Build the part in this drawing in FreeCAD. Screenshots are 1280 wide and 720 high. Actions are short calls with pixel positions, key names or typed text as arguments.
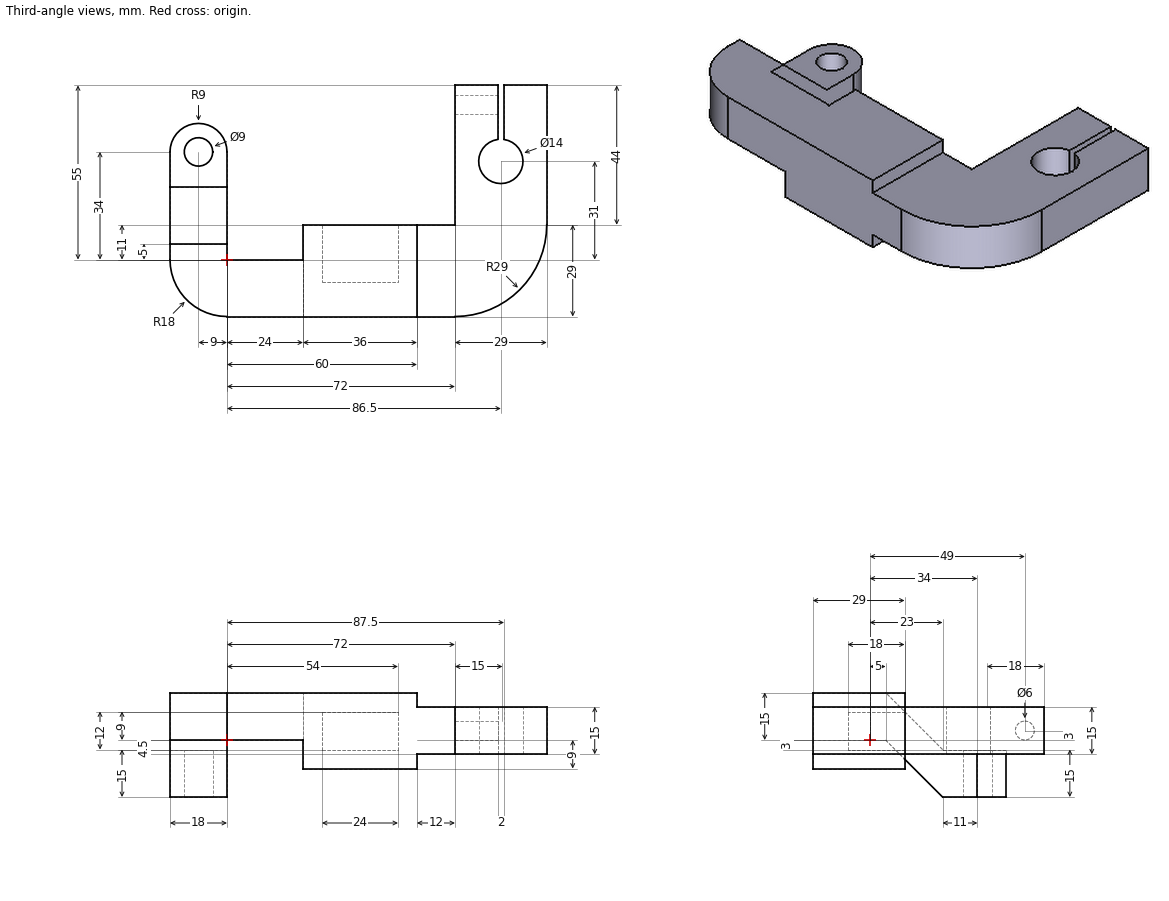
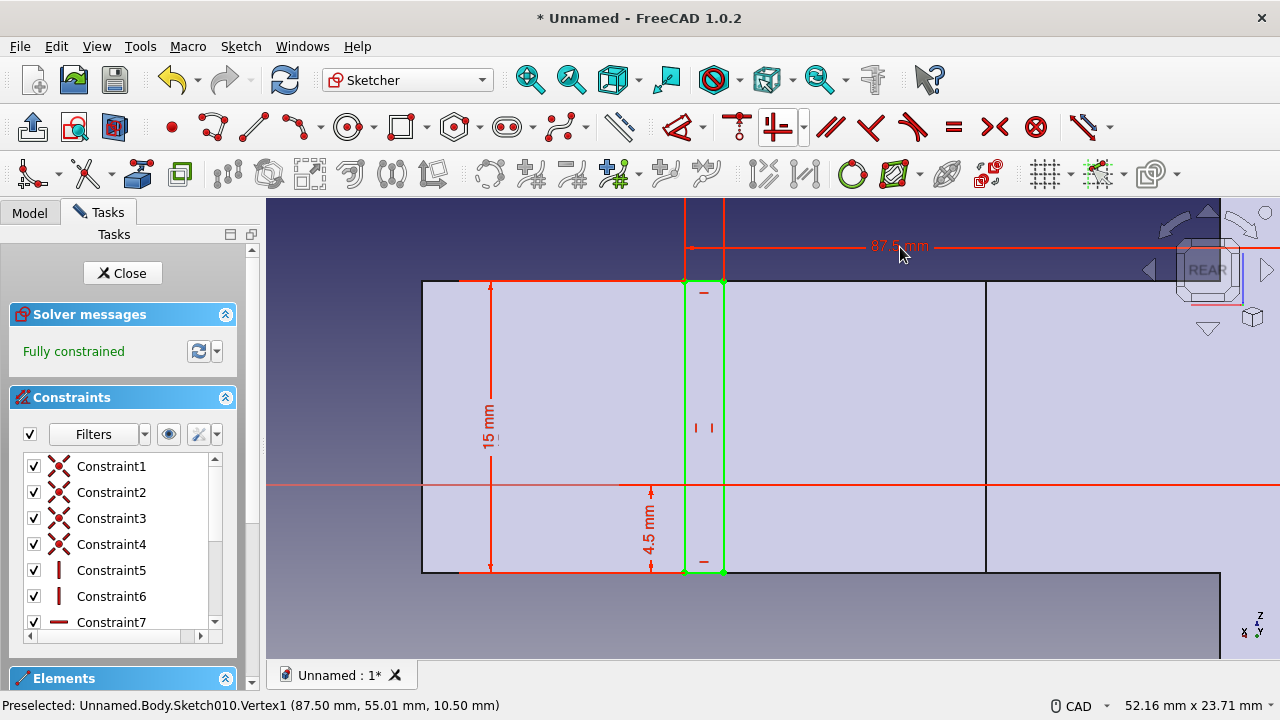
click(123, 273)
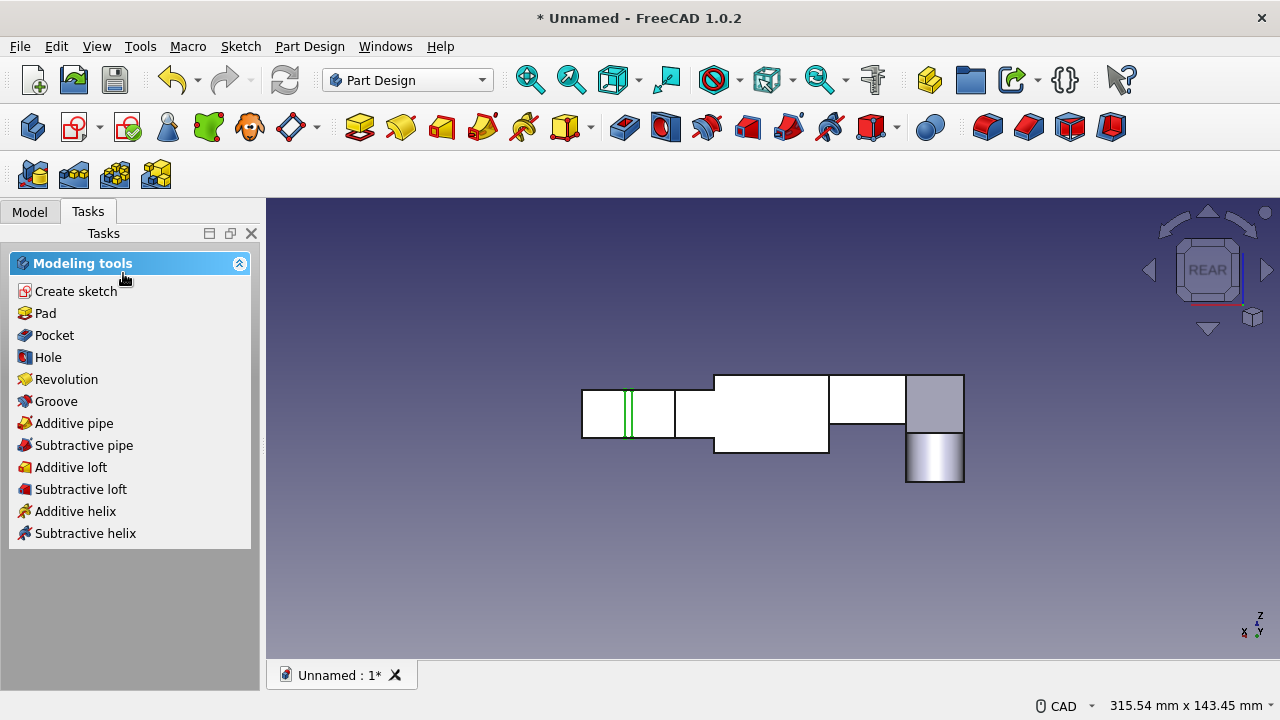
click(625, 128)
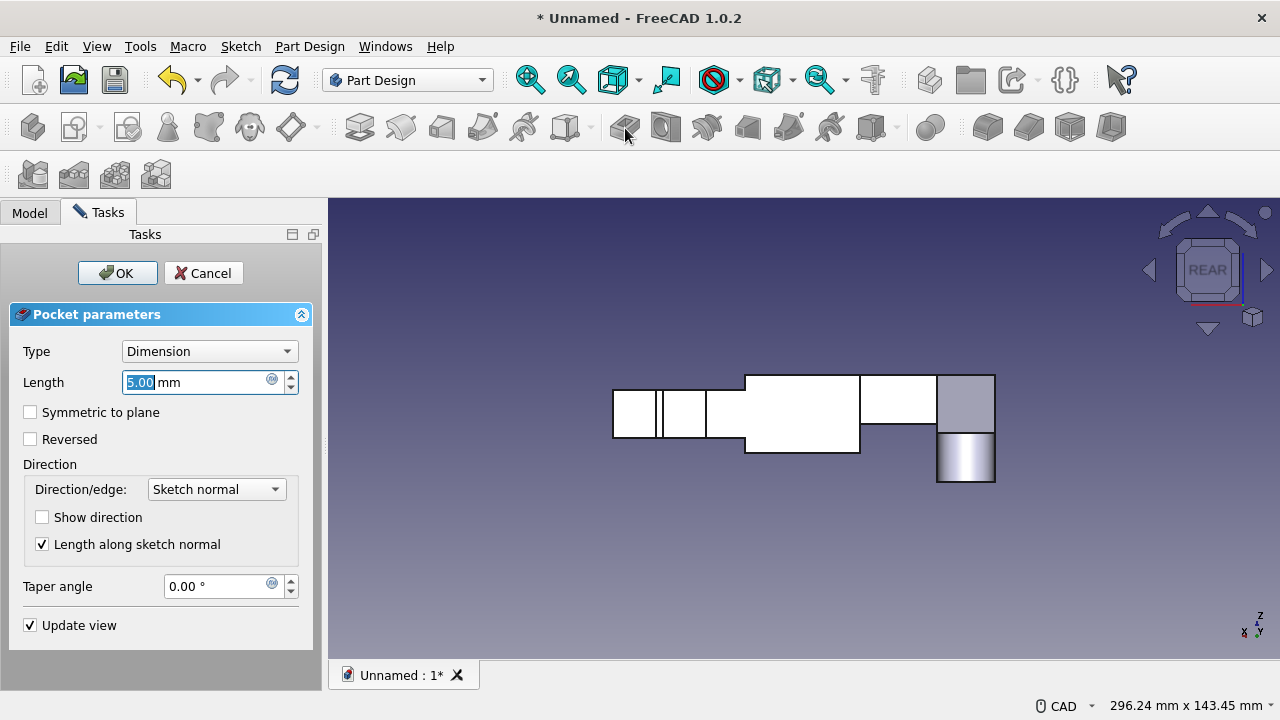
text(18)
key(Tab)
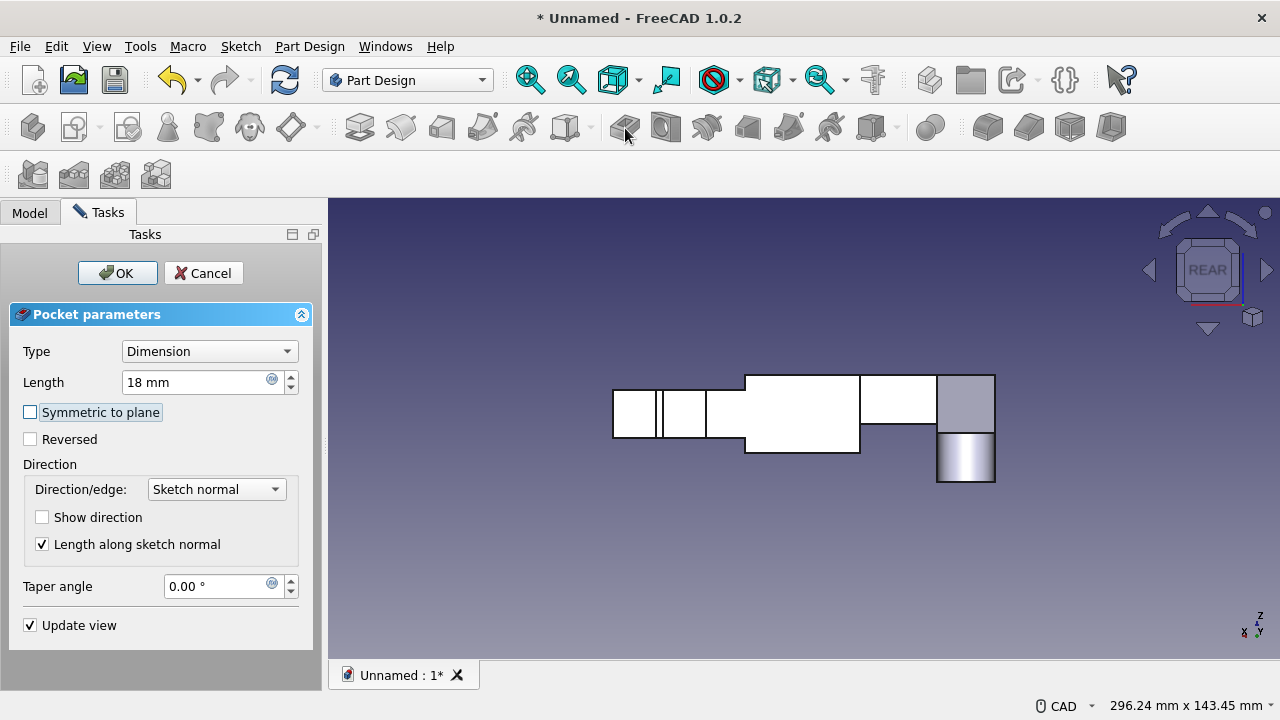
click(118, 273)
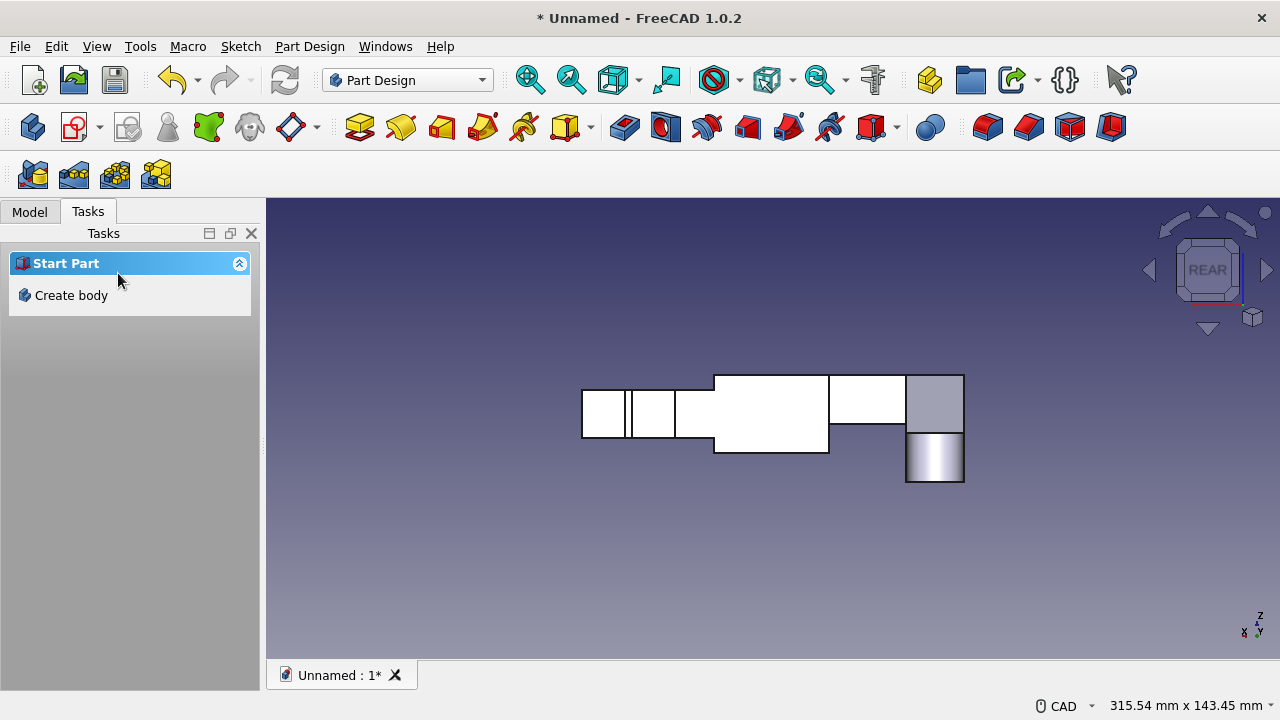
click(531, 80)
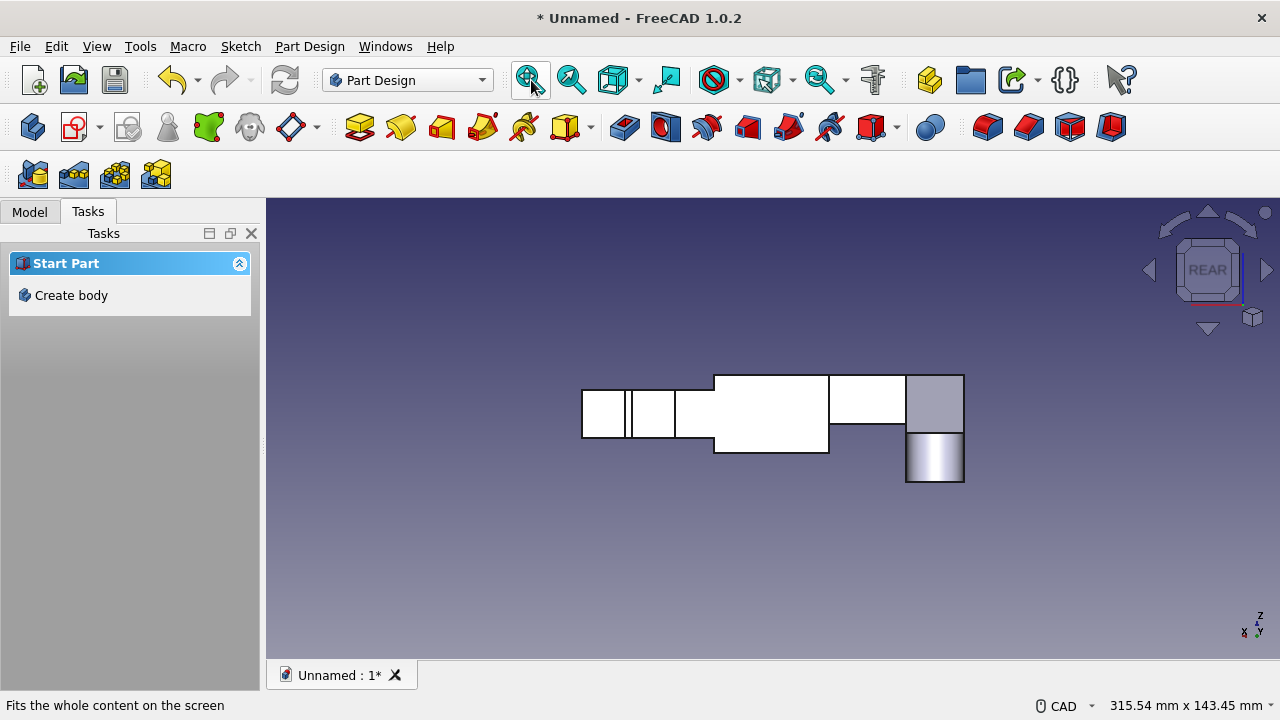
key(6)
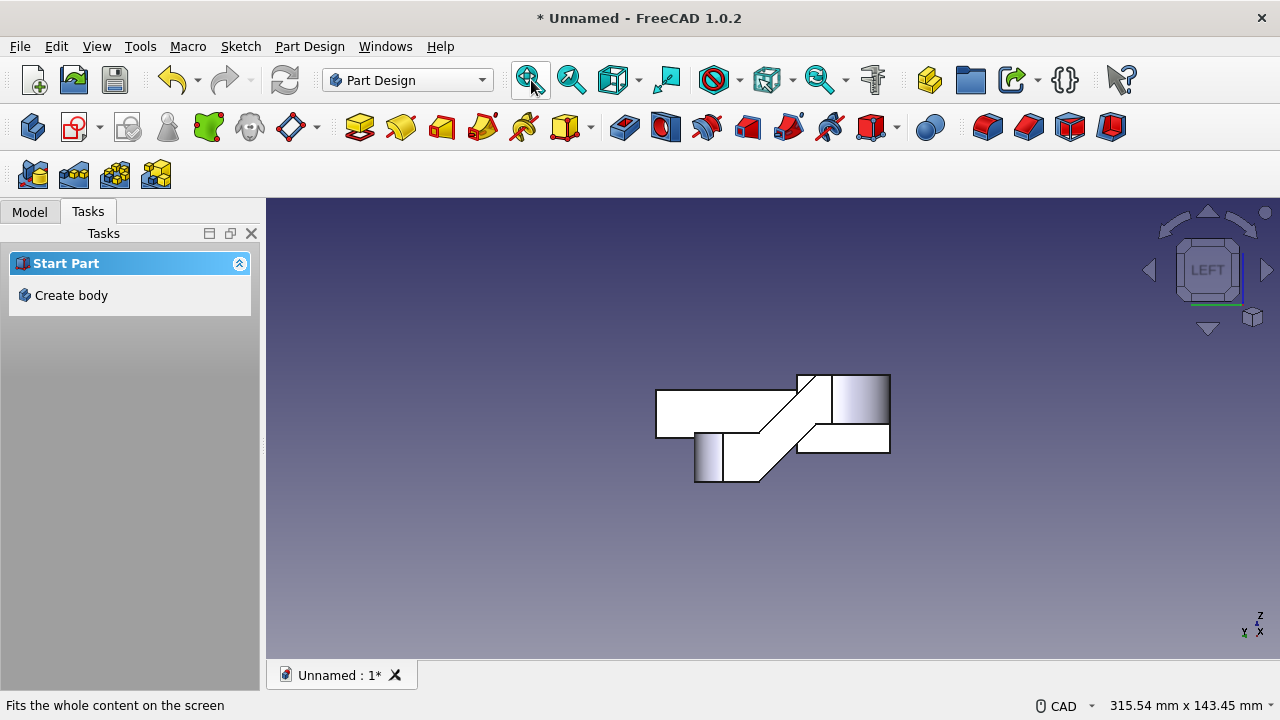
click(531, 80)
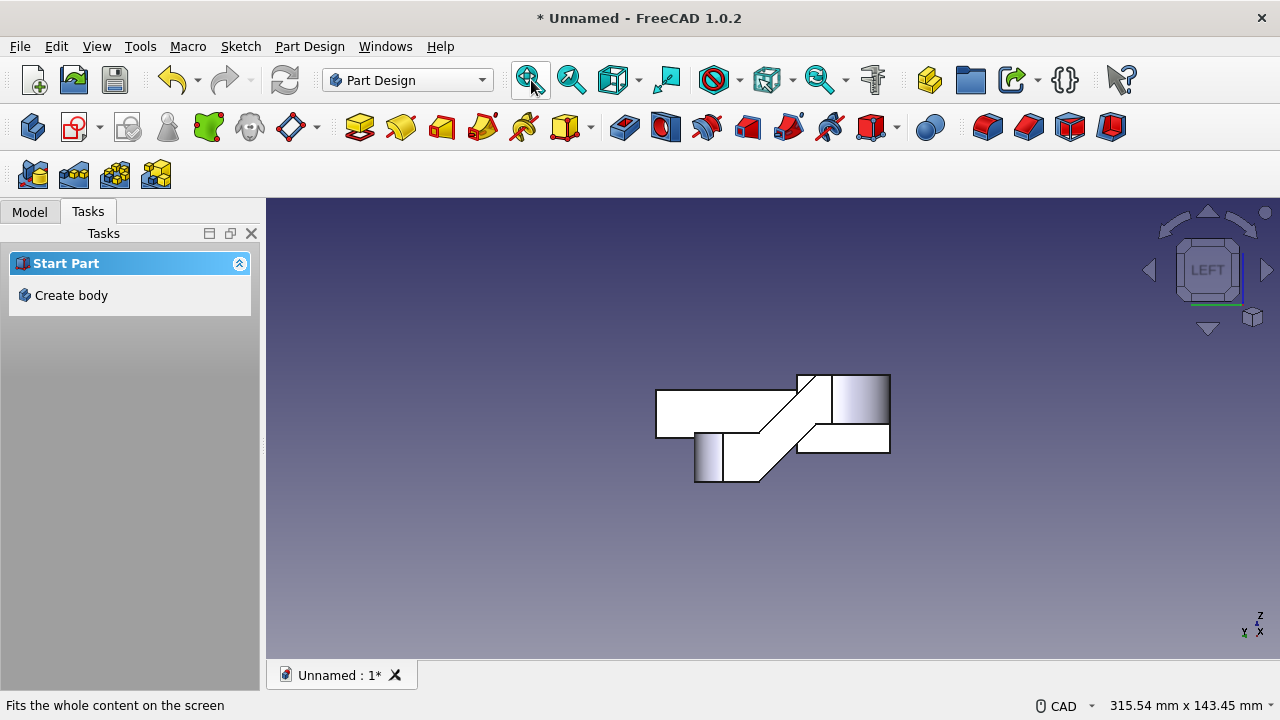
click(686, 413)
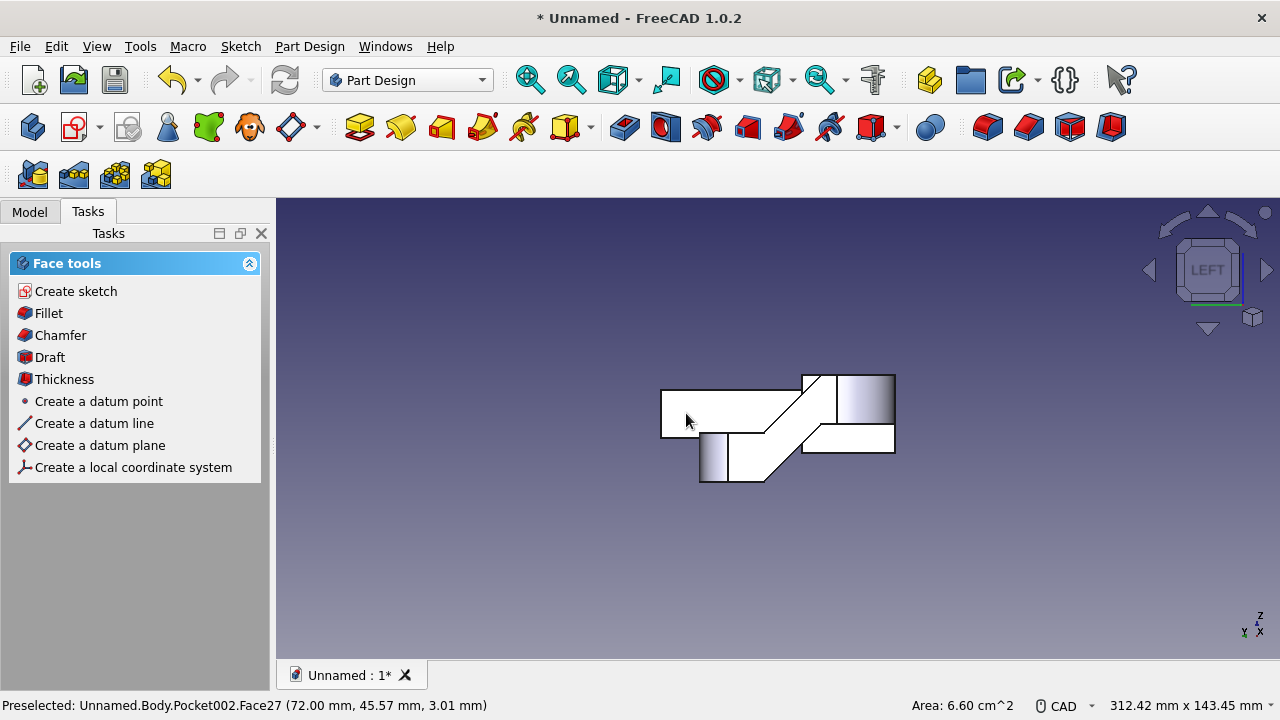
click(74, 128)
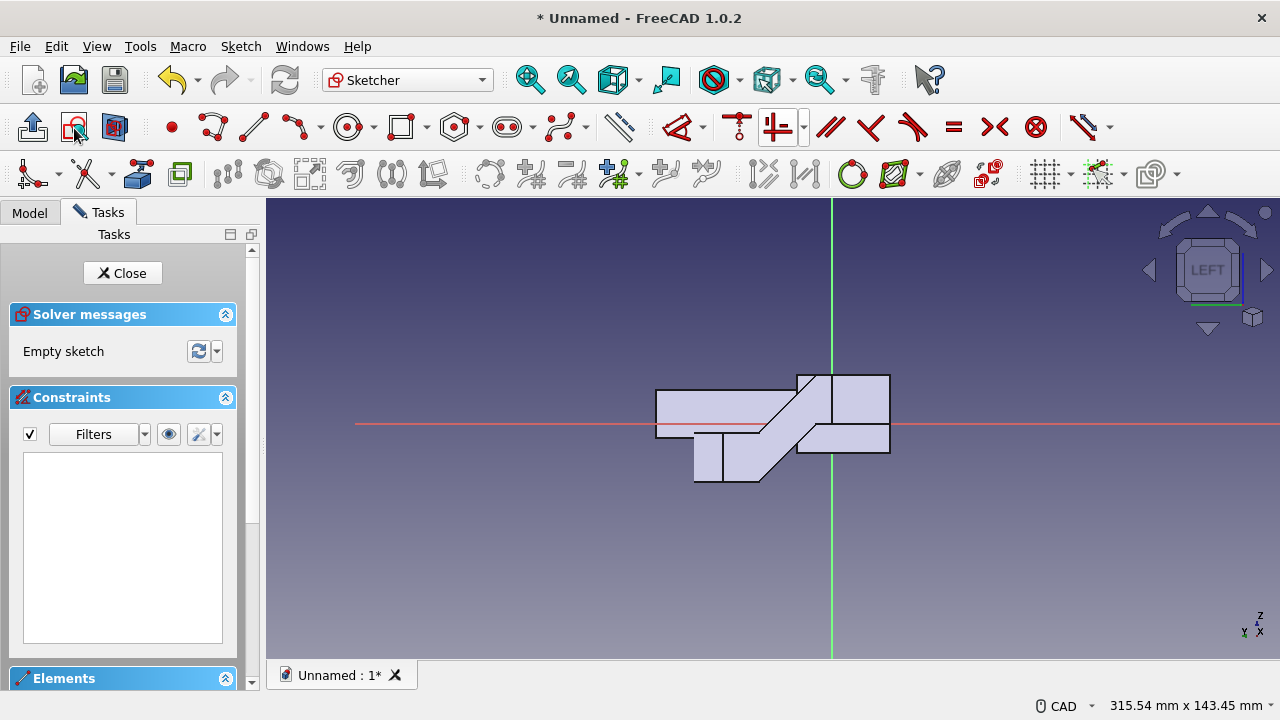
click(115, 128)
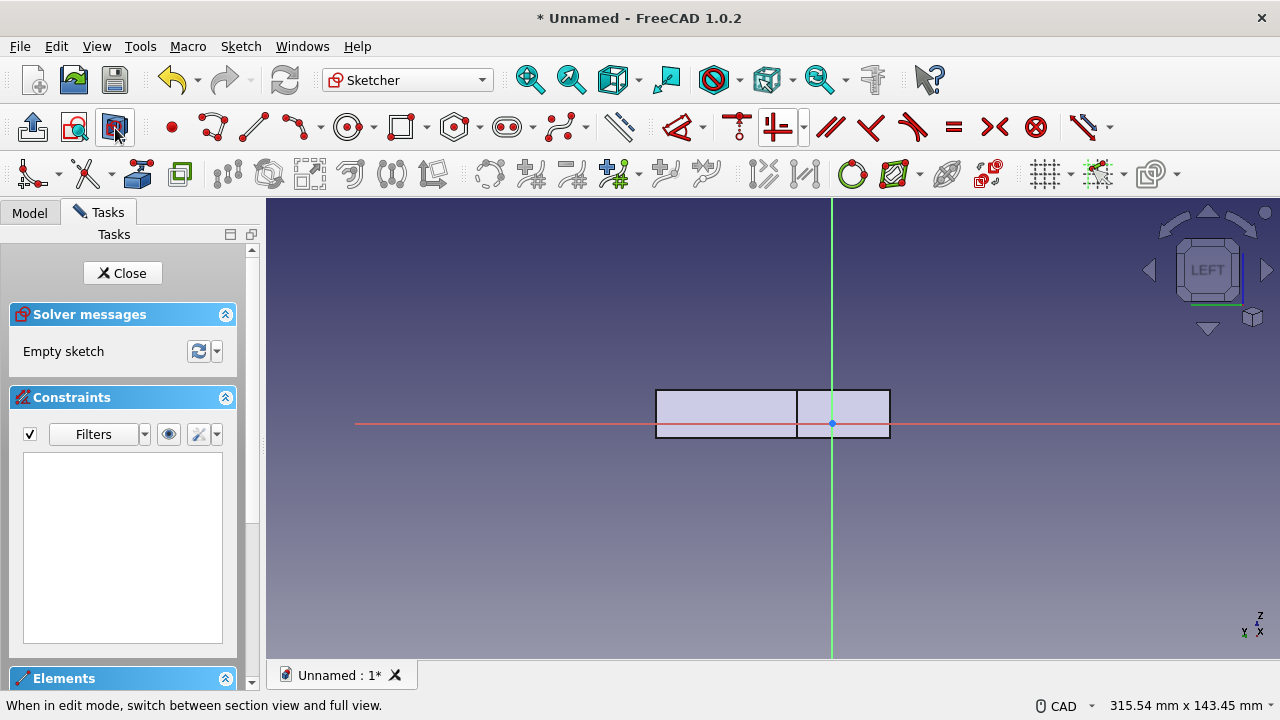
scroll(673, 413, up, 13)